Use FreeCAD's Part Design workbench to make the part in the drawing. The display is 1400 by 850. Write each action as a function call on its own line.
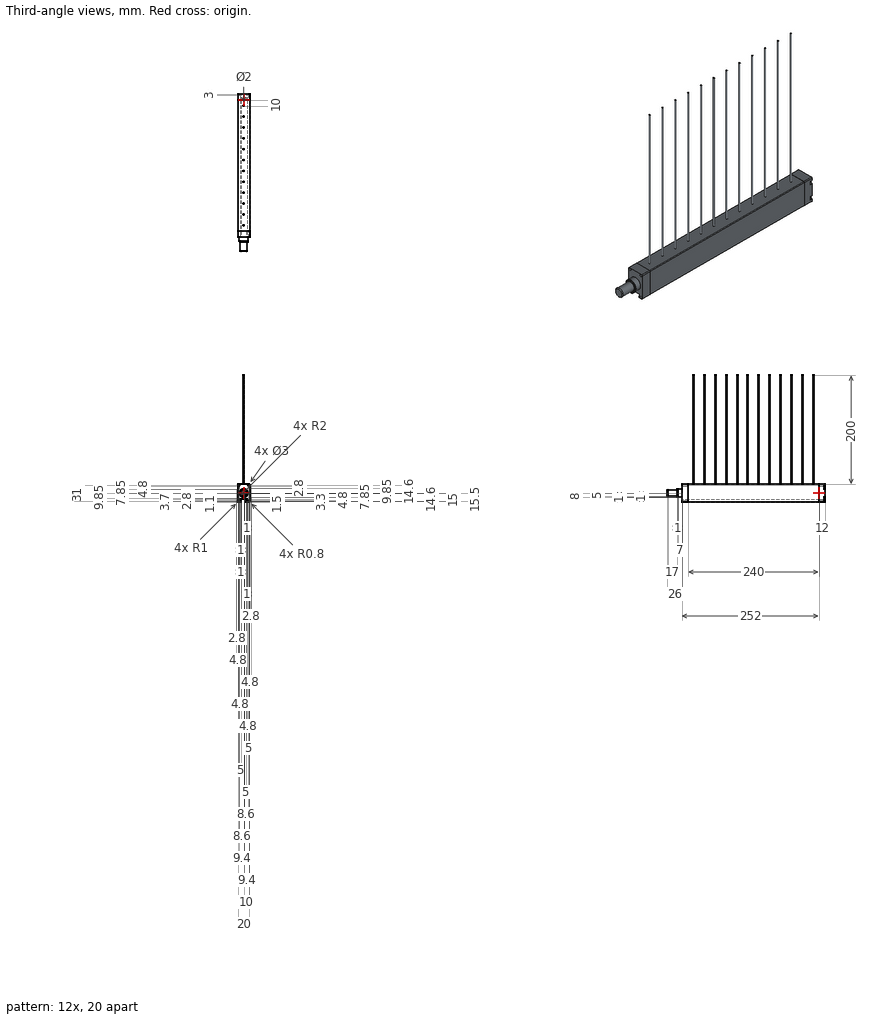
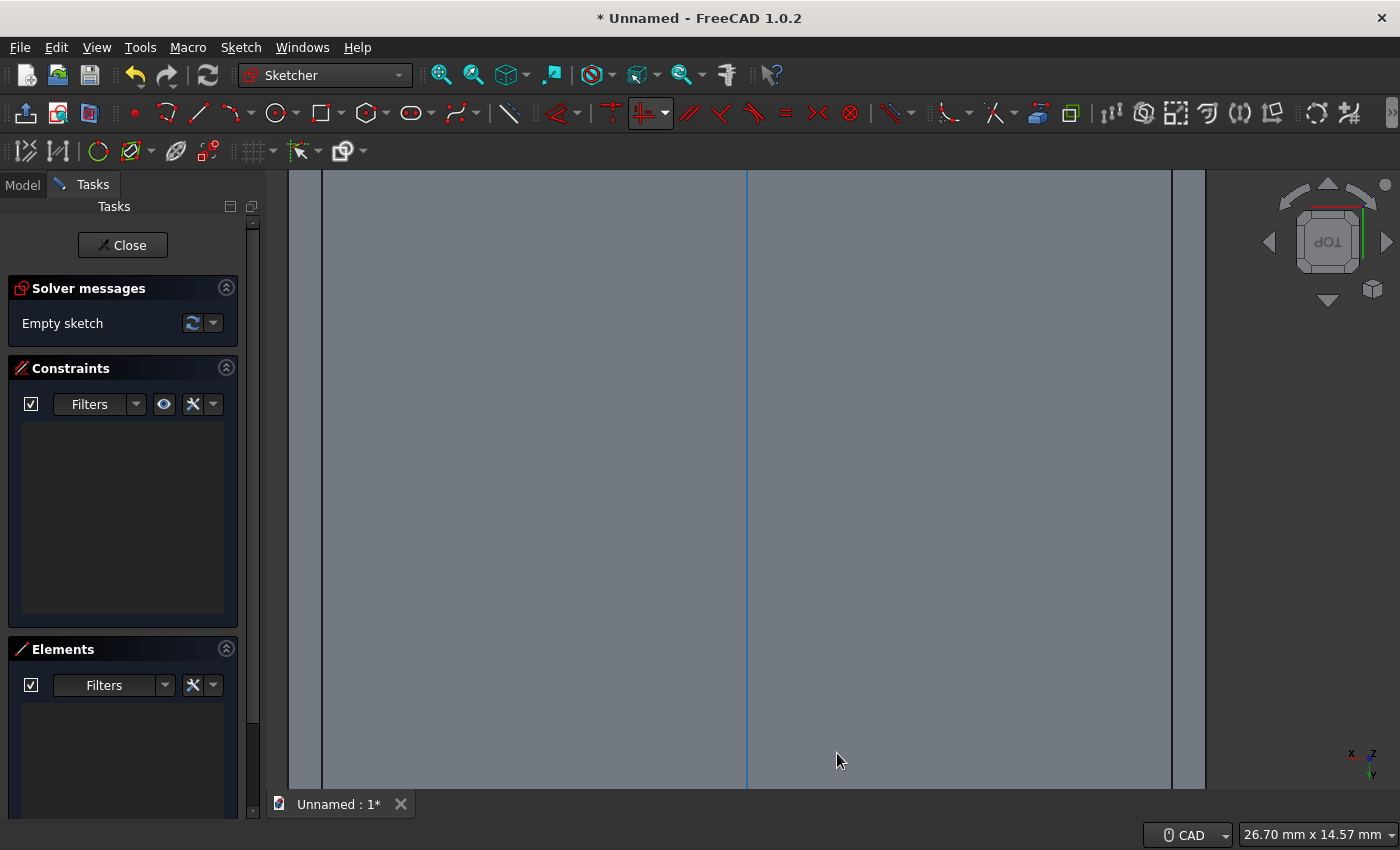
scroll(743, 463, up, 8)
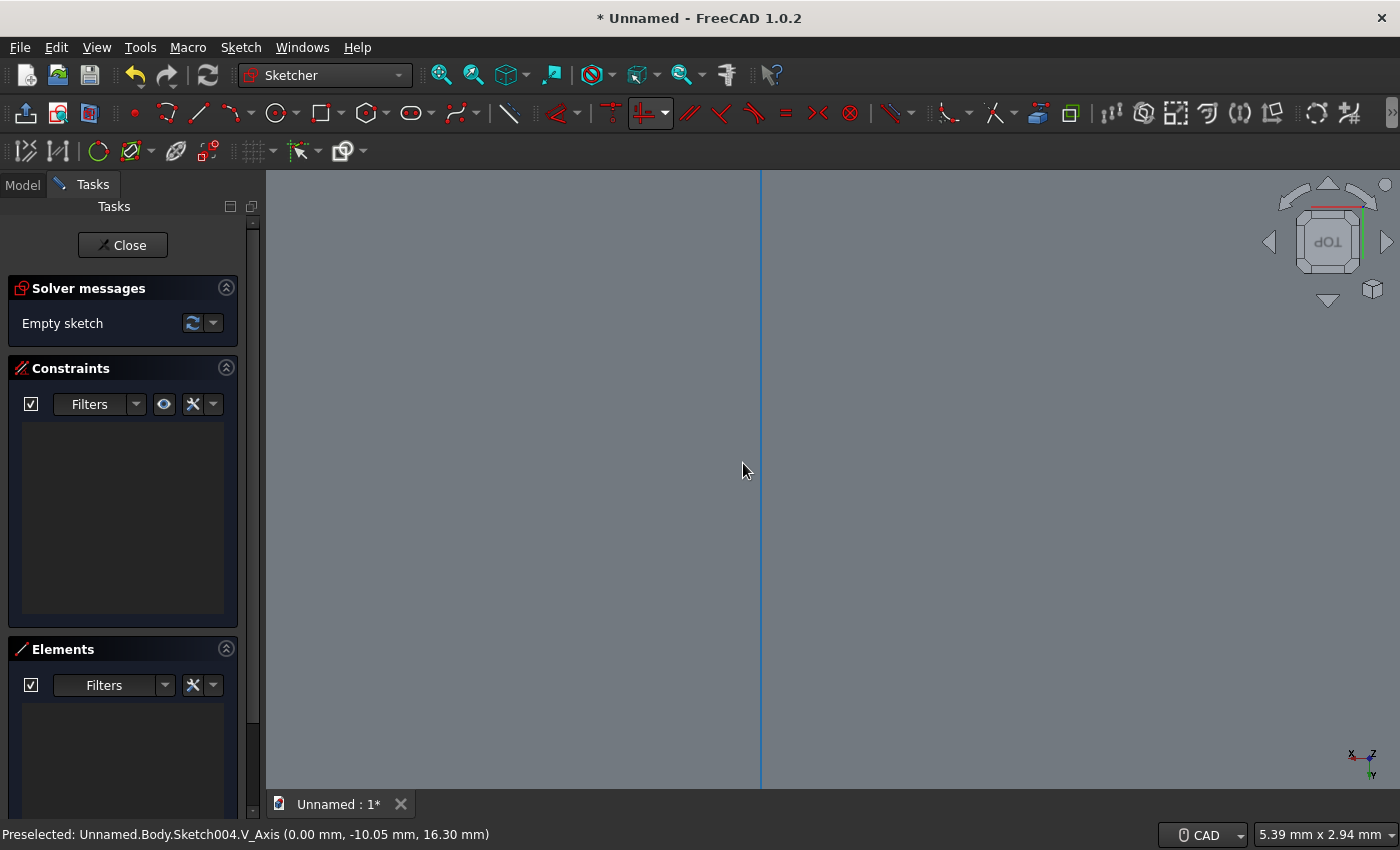
click(276, 114)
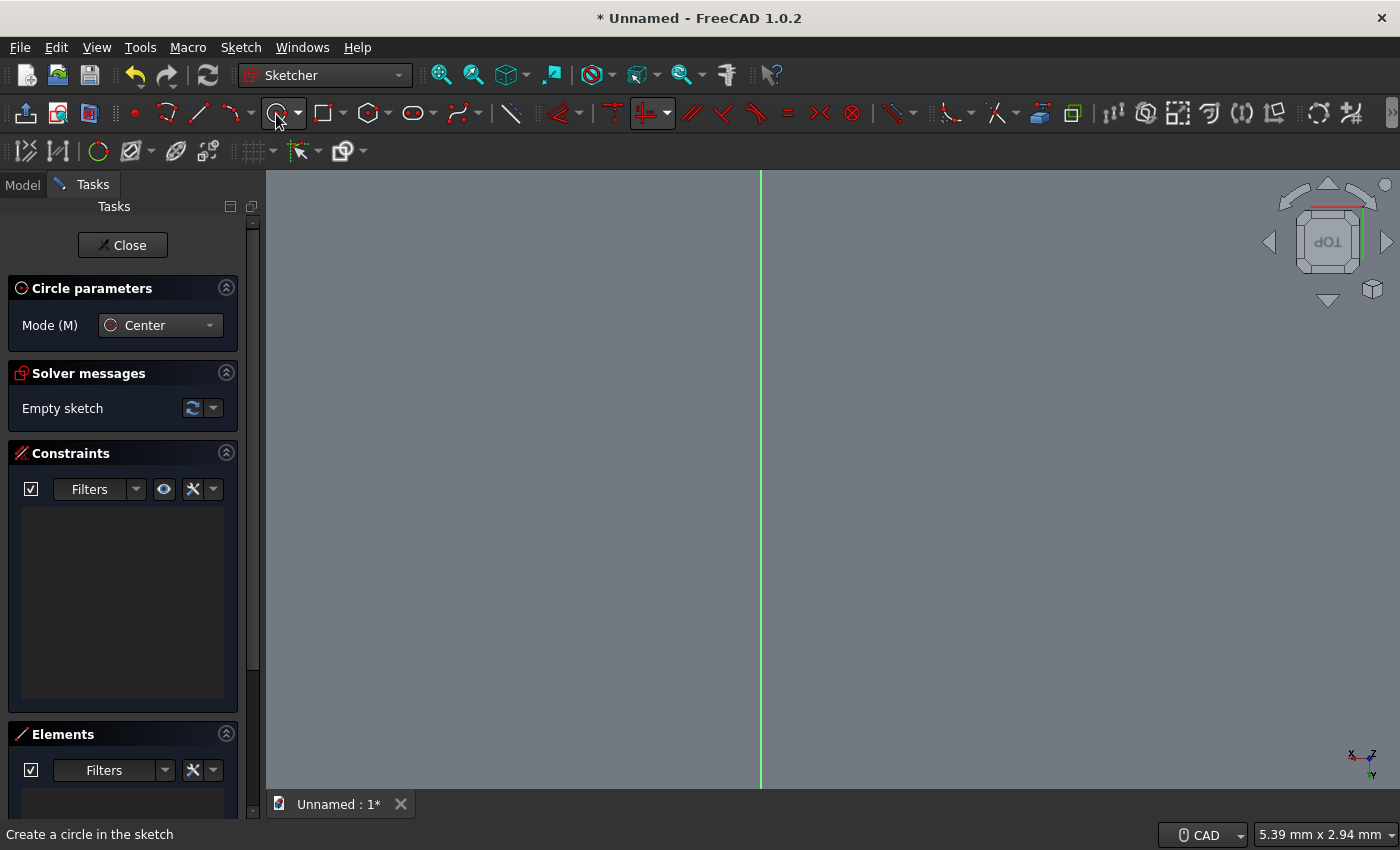
click(761, 477)
click(910, 328)
key(Escape)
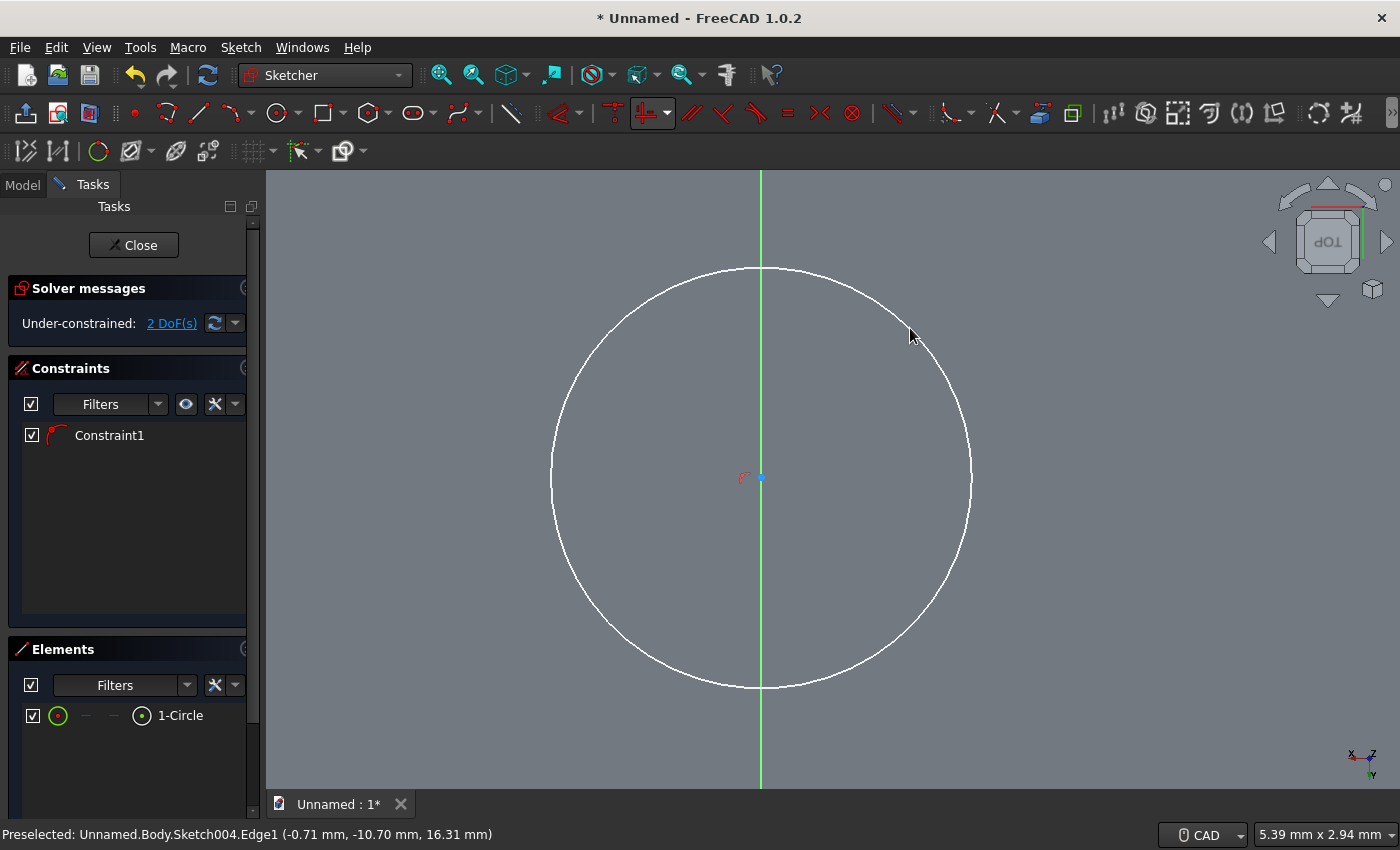
click(558, 114)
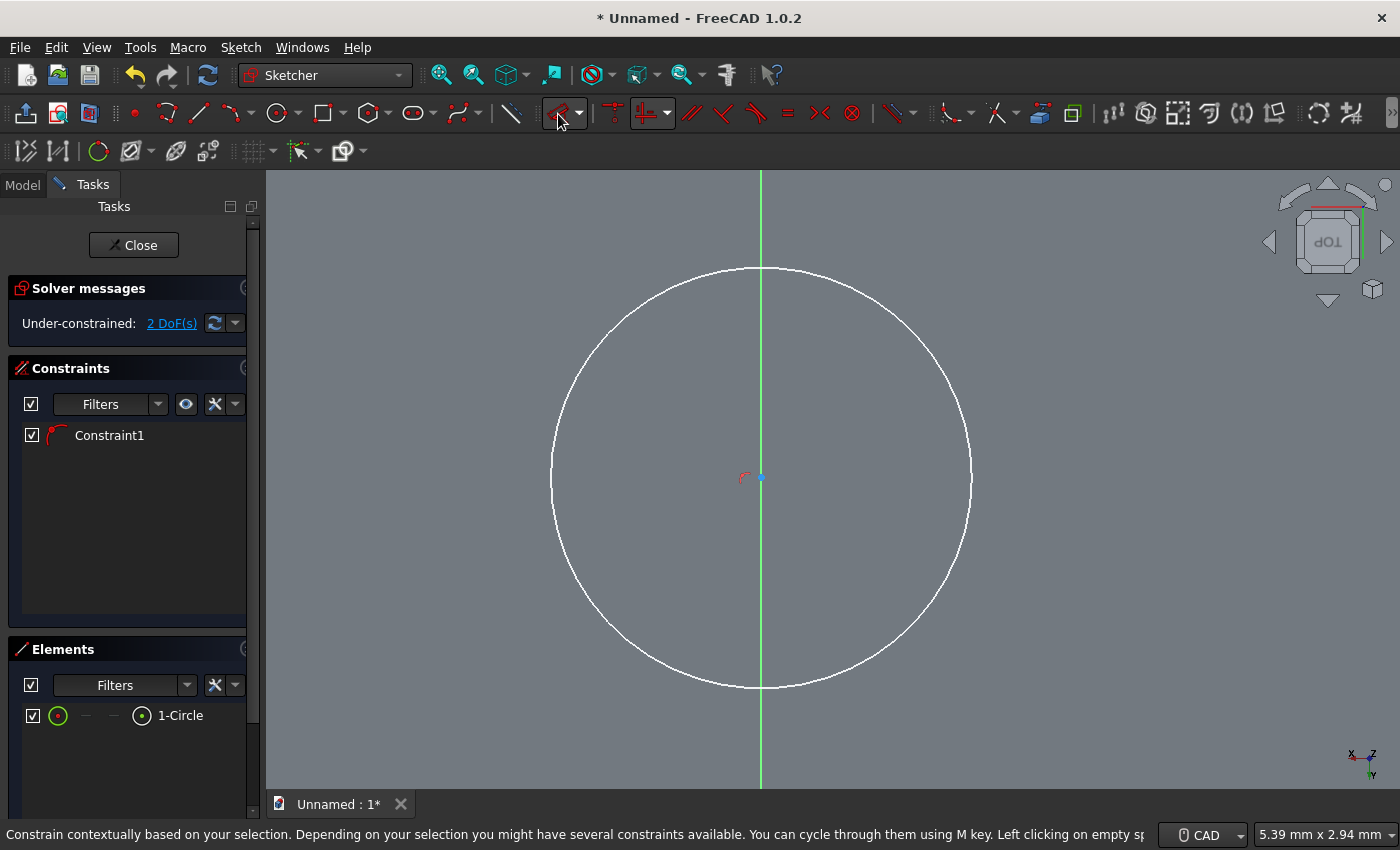
click(910, 329)
click(933, 306)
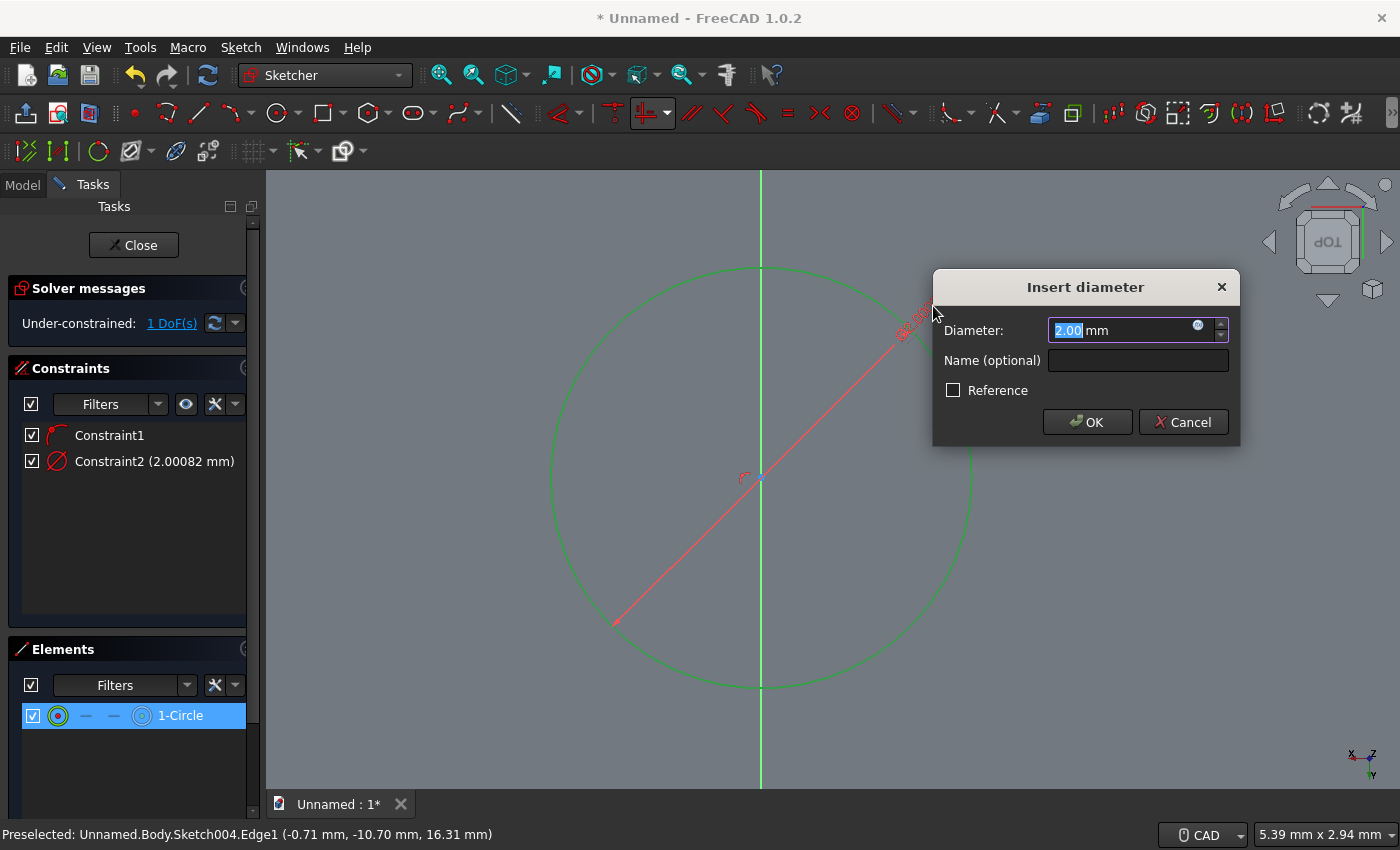
text(2)
key(Return)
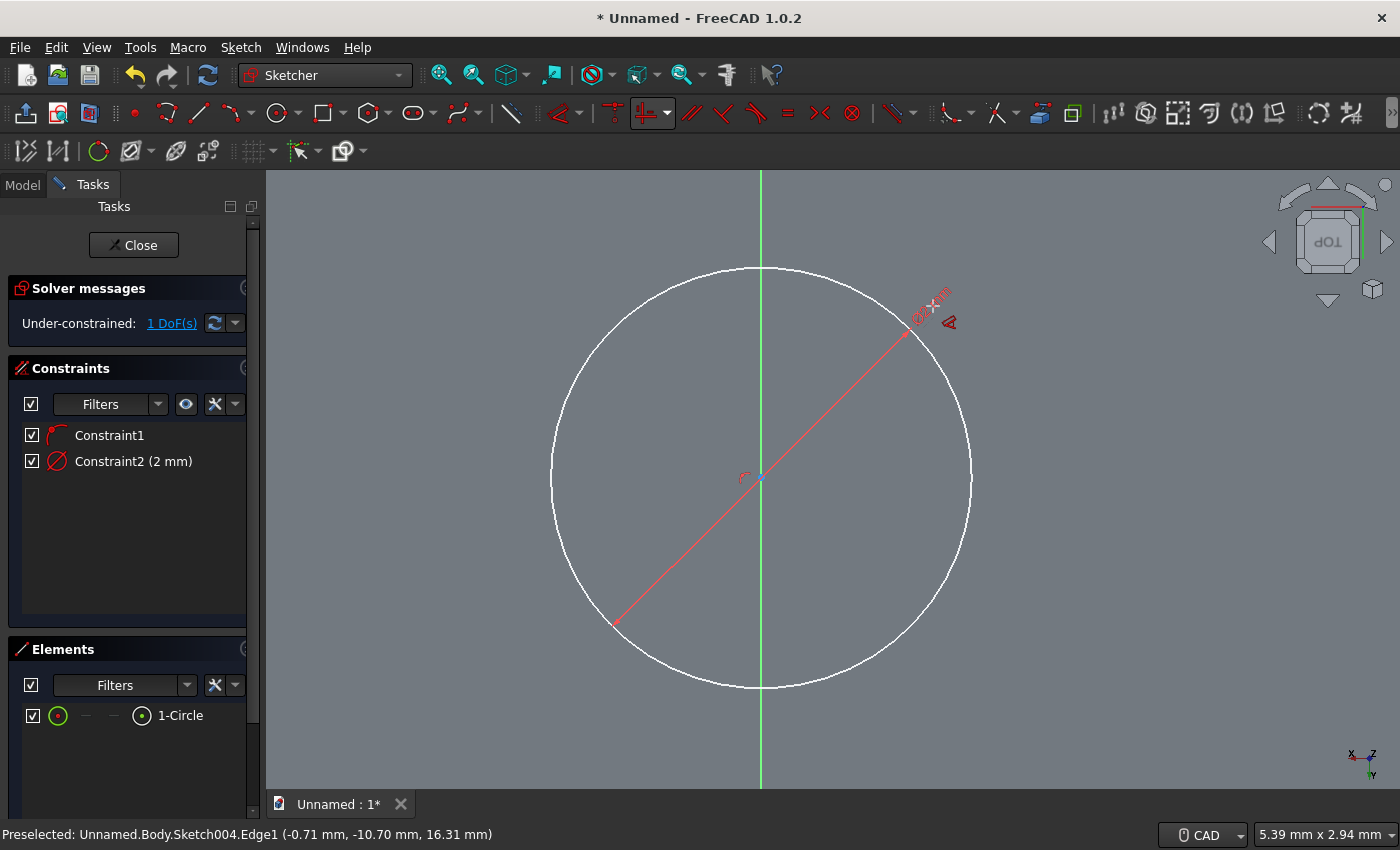
click(761, 478)
click(795, 619)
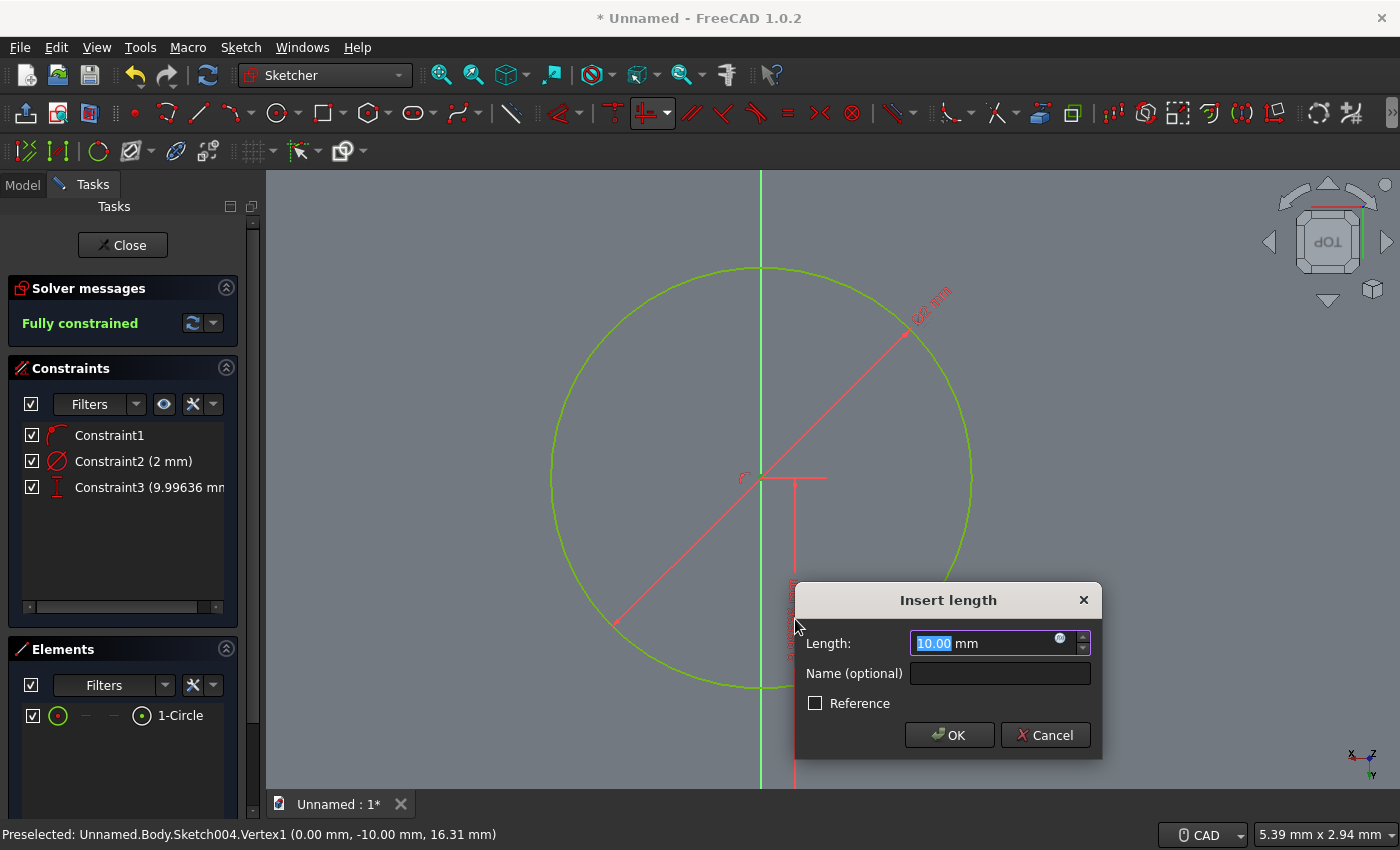
text(10)
key(Return)
key(Escape)